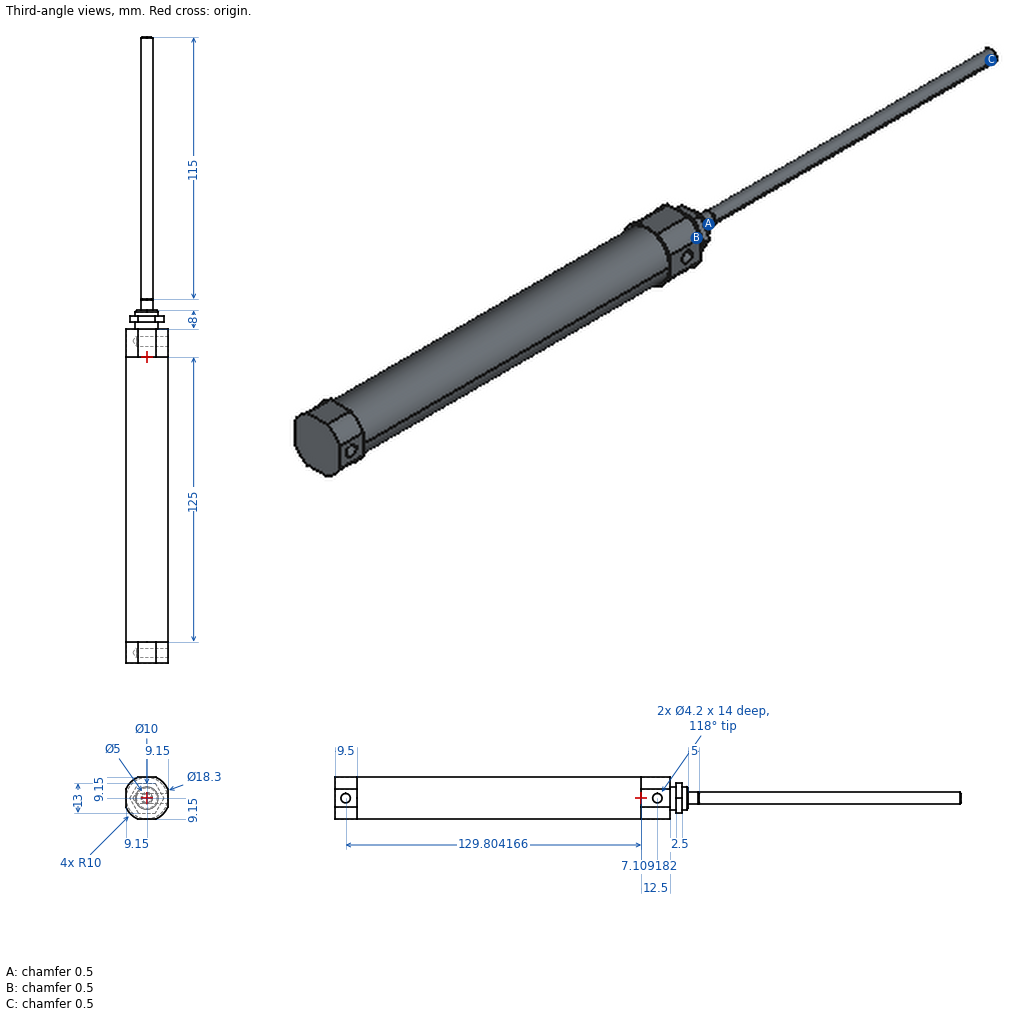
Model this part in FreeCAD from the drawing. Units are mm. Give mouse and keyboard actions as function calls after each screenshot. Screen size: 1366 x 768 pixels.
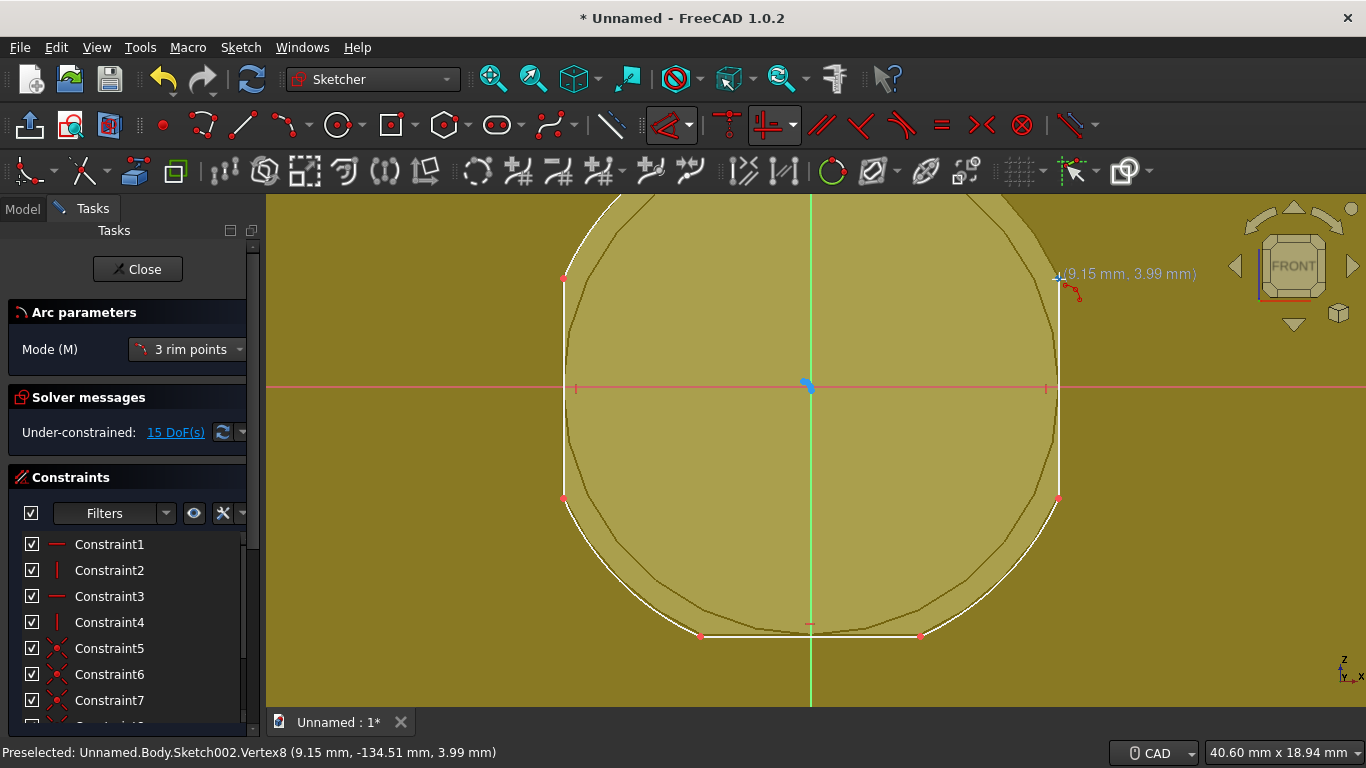
scroll(619, 580, down, 2)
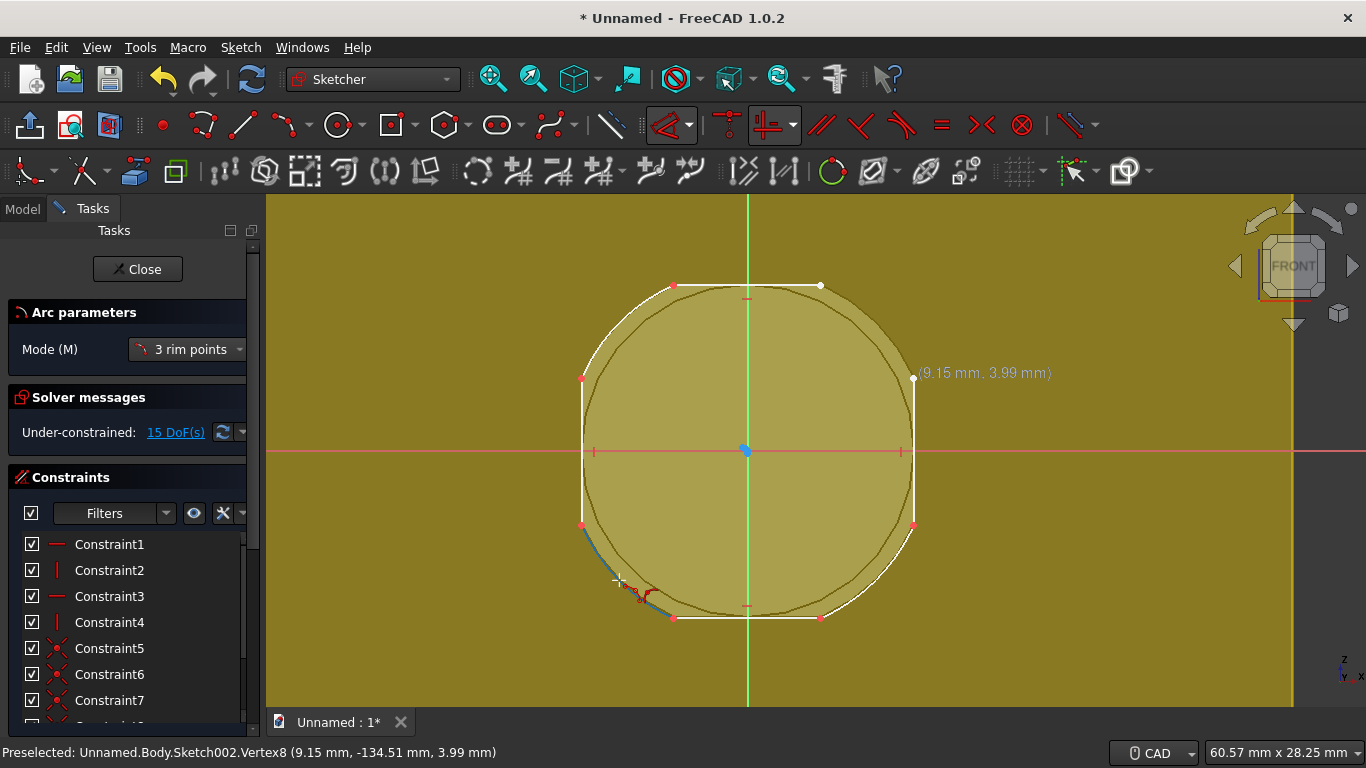
click(821, 285)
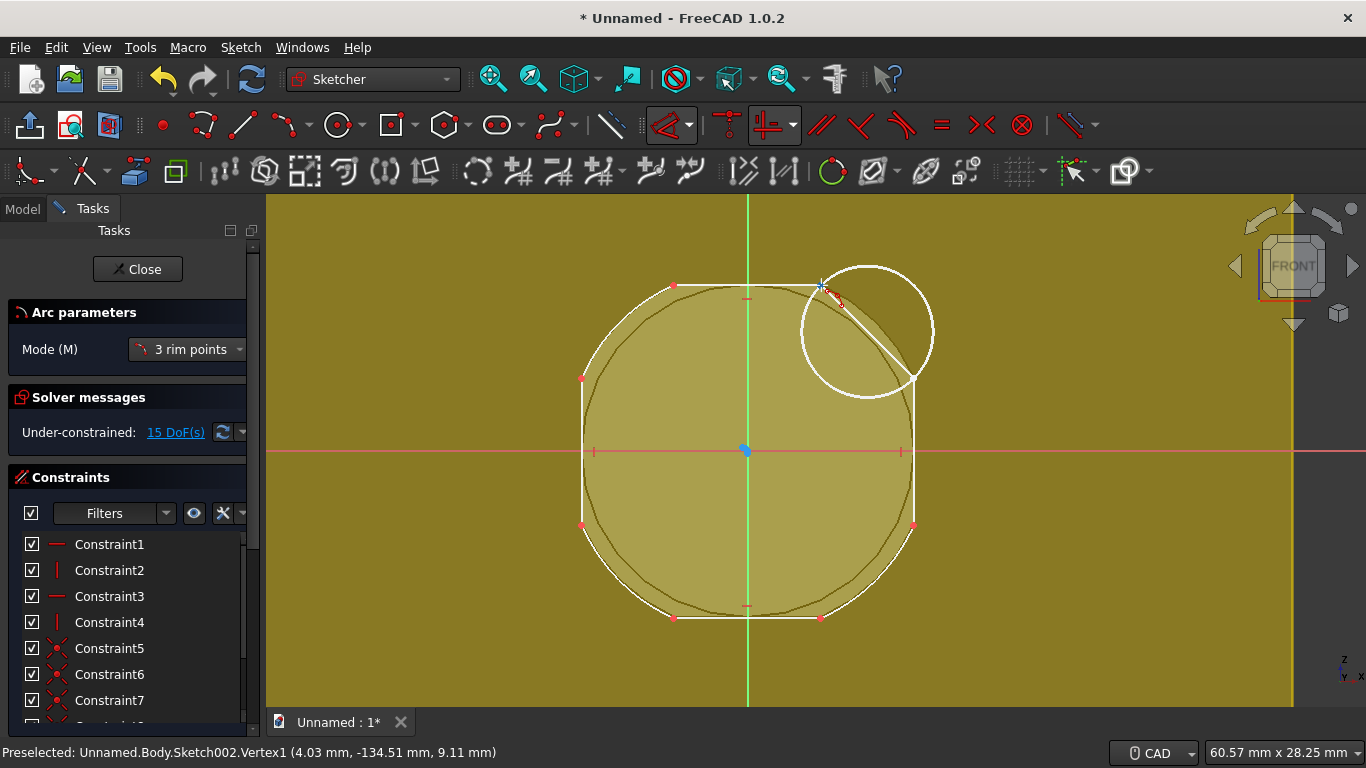
scroll(876, 322, up, 2)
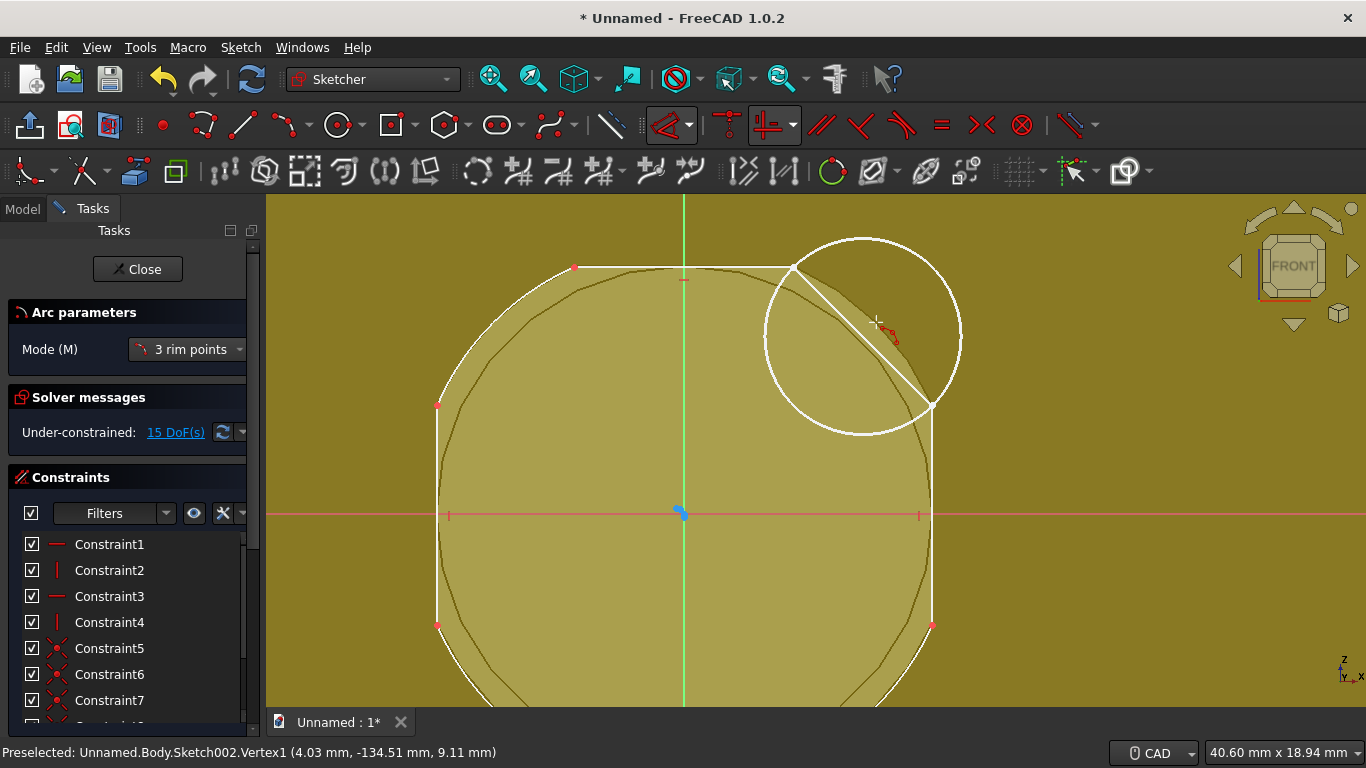
click(876, 322)
key(Escape)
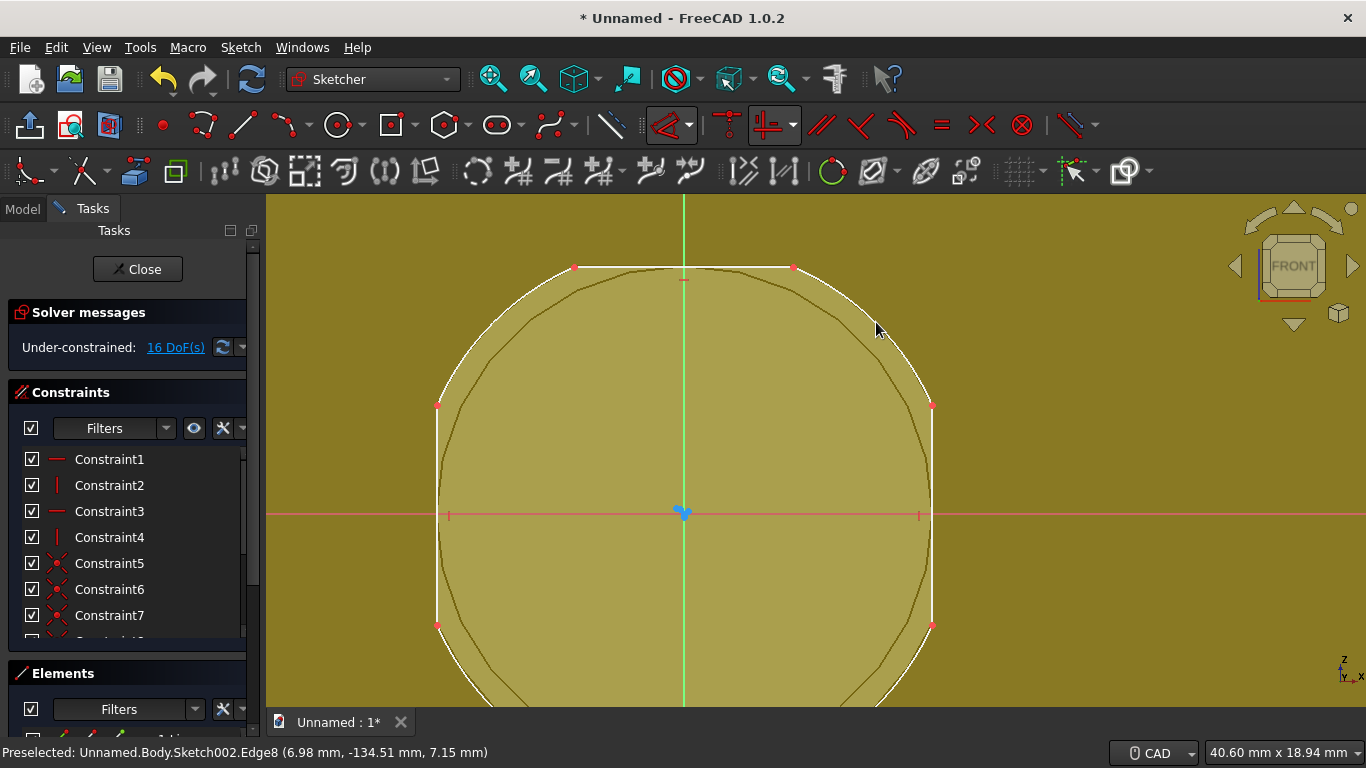
click(523, 297)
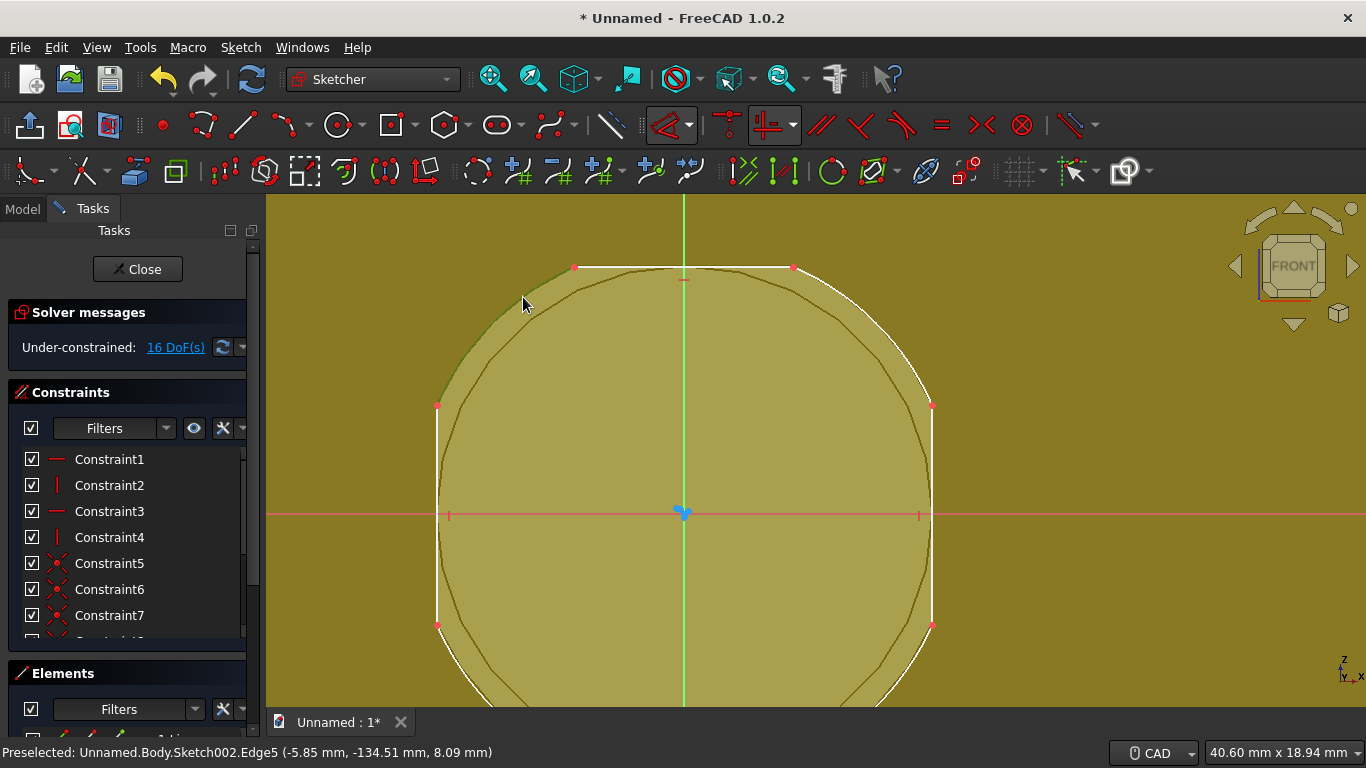
click(467, 677)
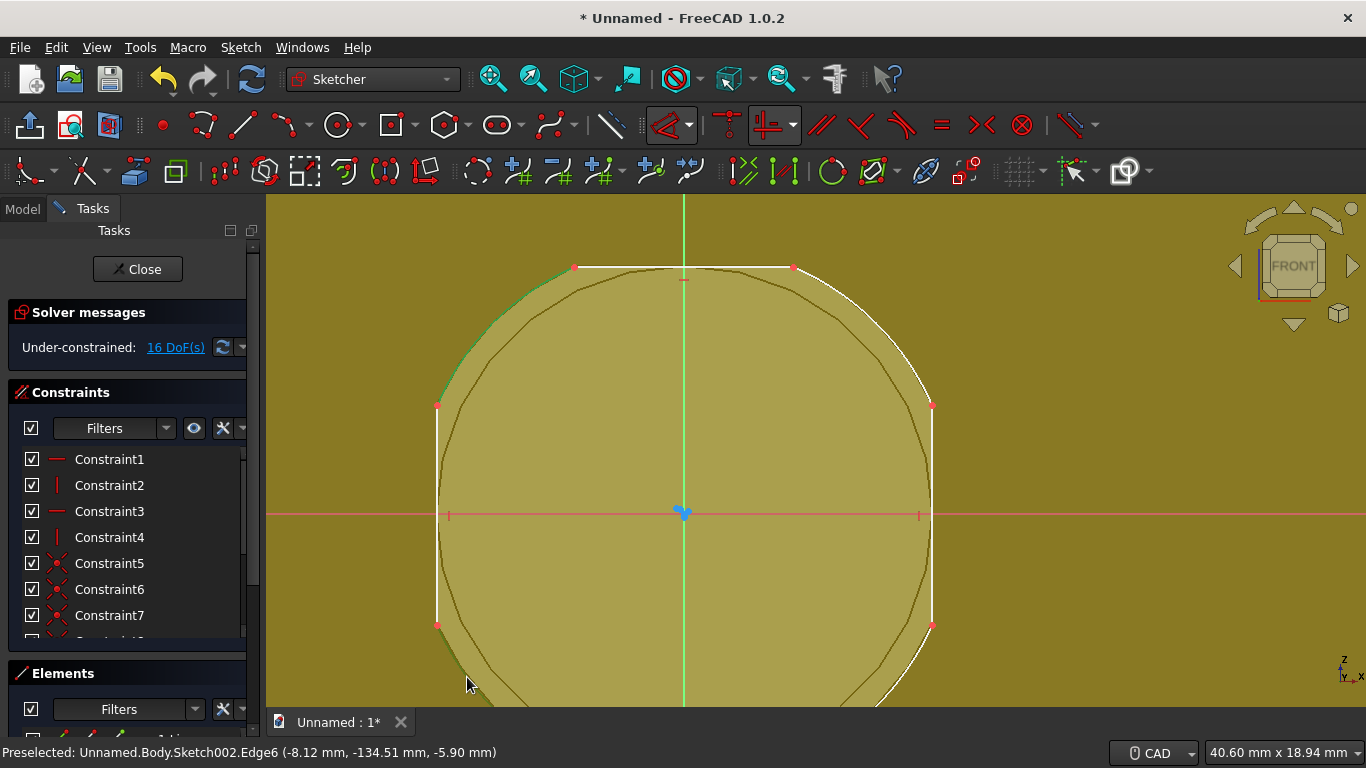
click(728, 126)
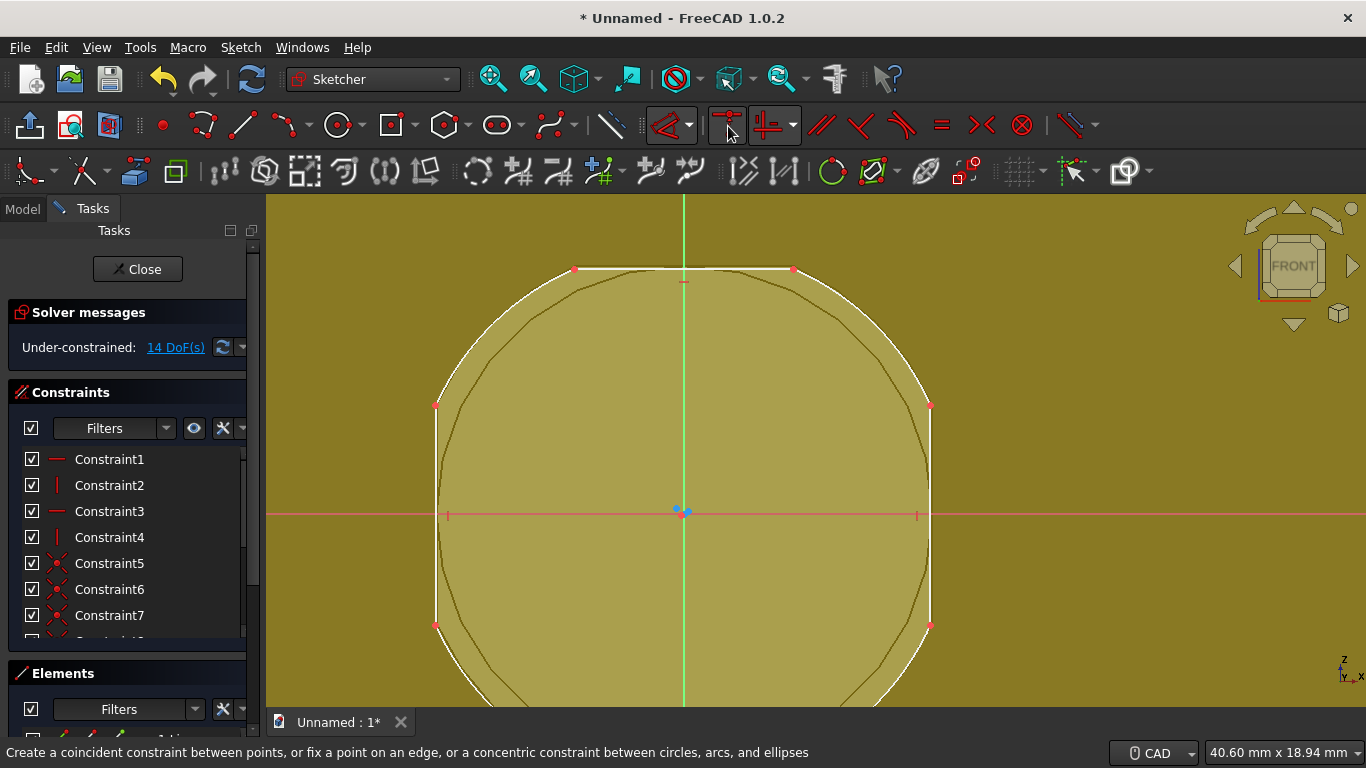
click(523, 299)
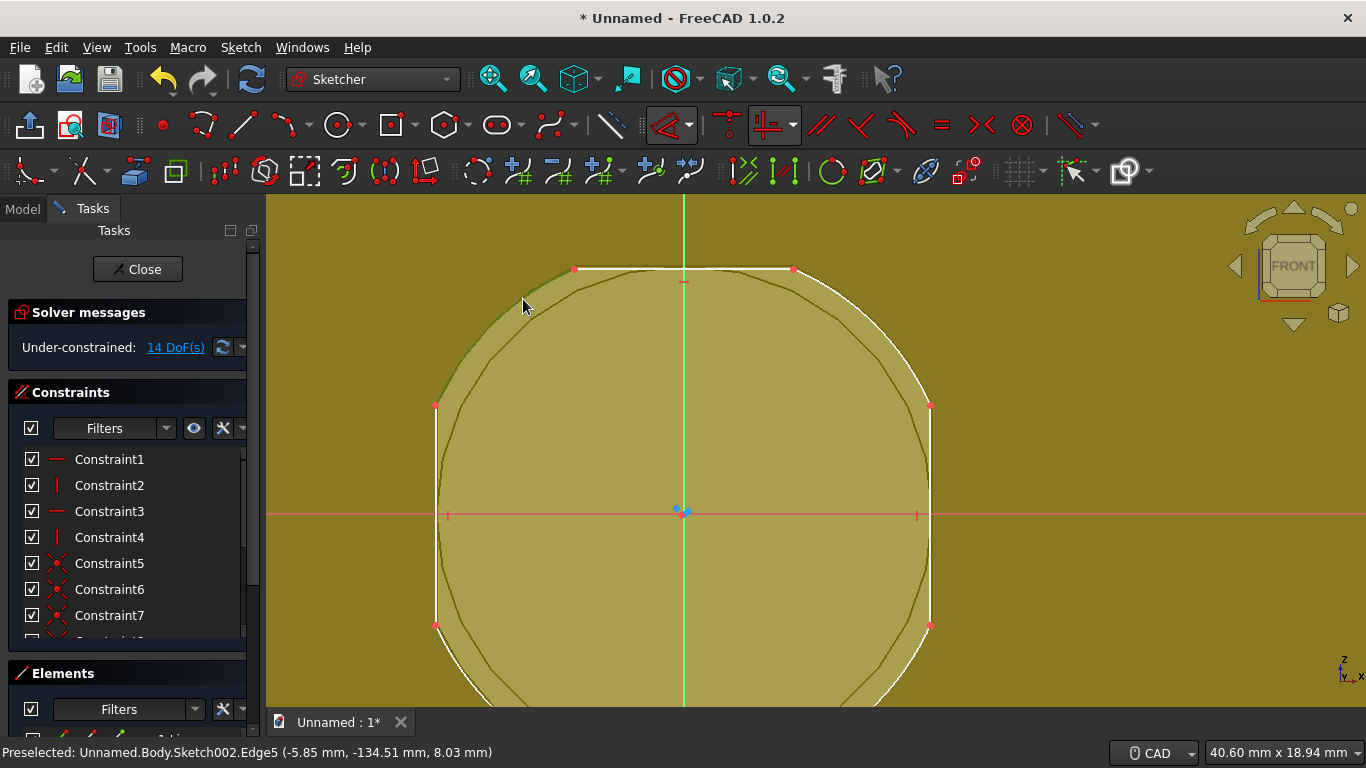
click(900, 676)